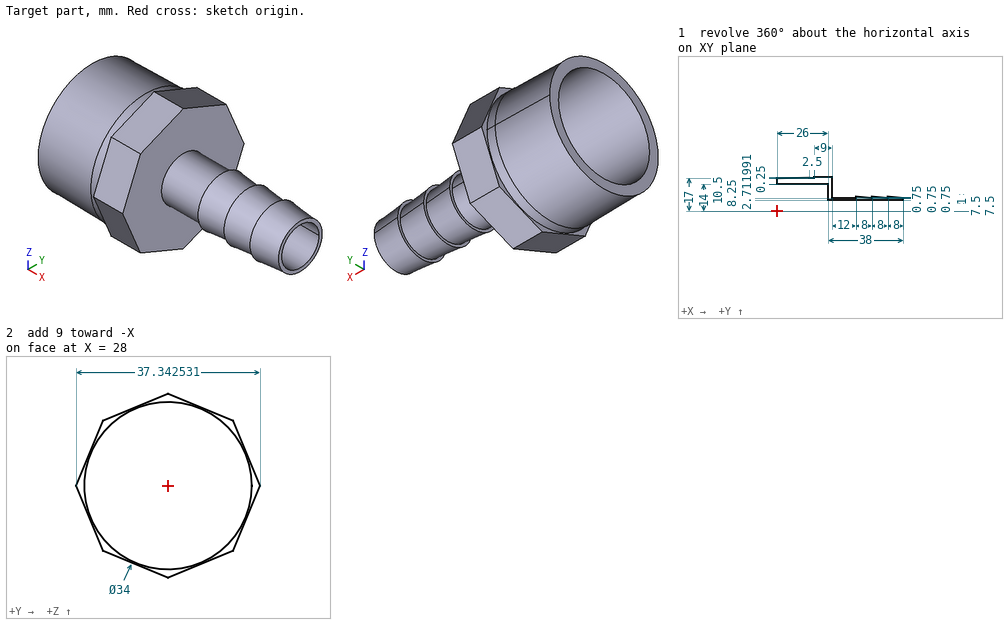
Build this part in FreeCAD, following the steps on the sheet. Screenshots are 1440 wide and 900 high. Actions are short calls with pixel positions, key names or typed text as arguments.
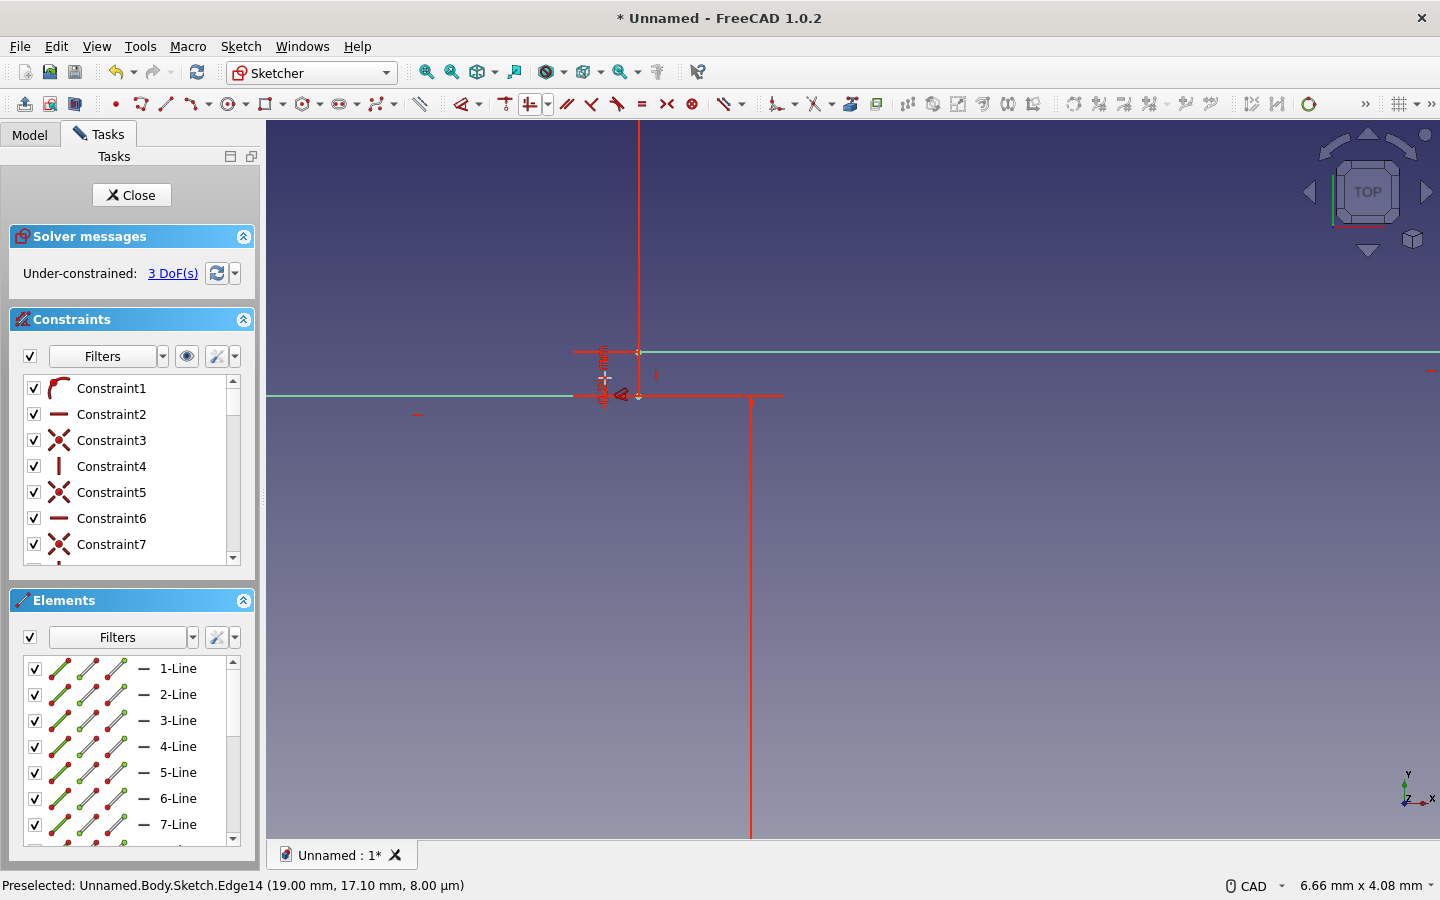
scroll(645, 389, down, 14)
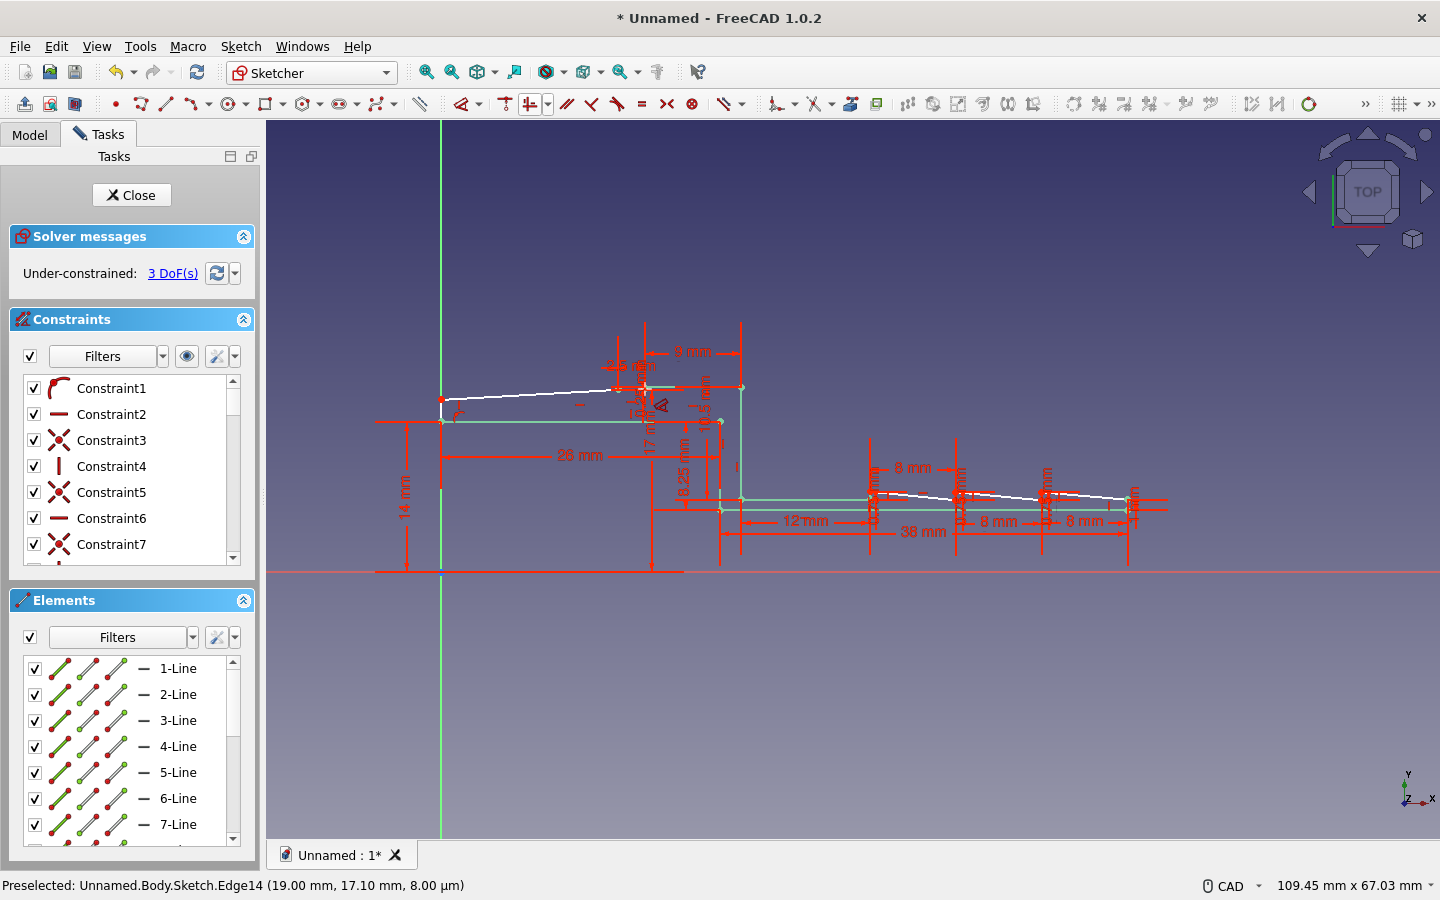
scroll(1042, 492, up, 3)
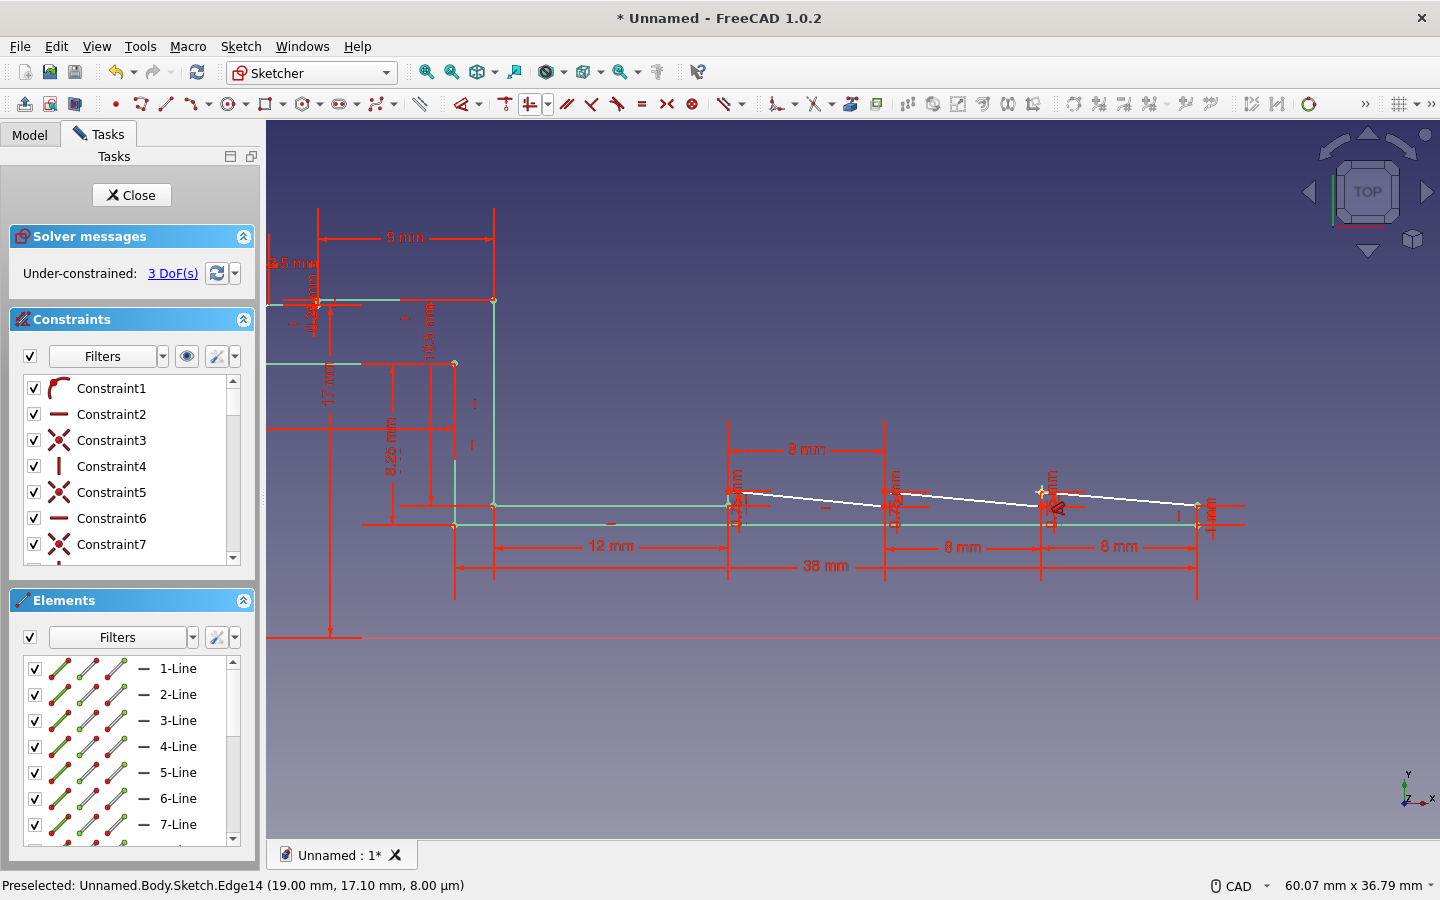
click(1041, 492)
click(1075, 598)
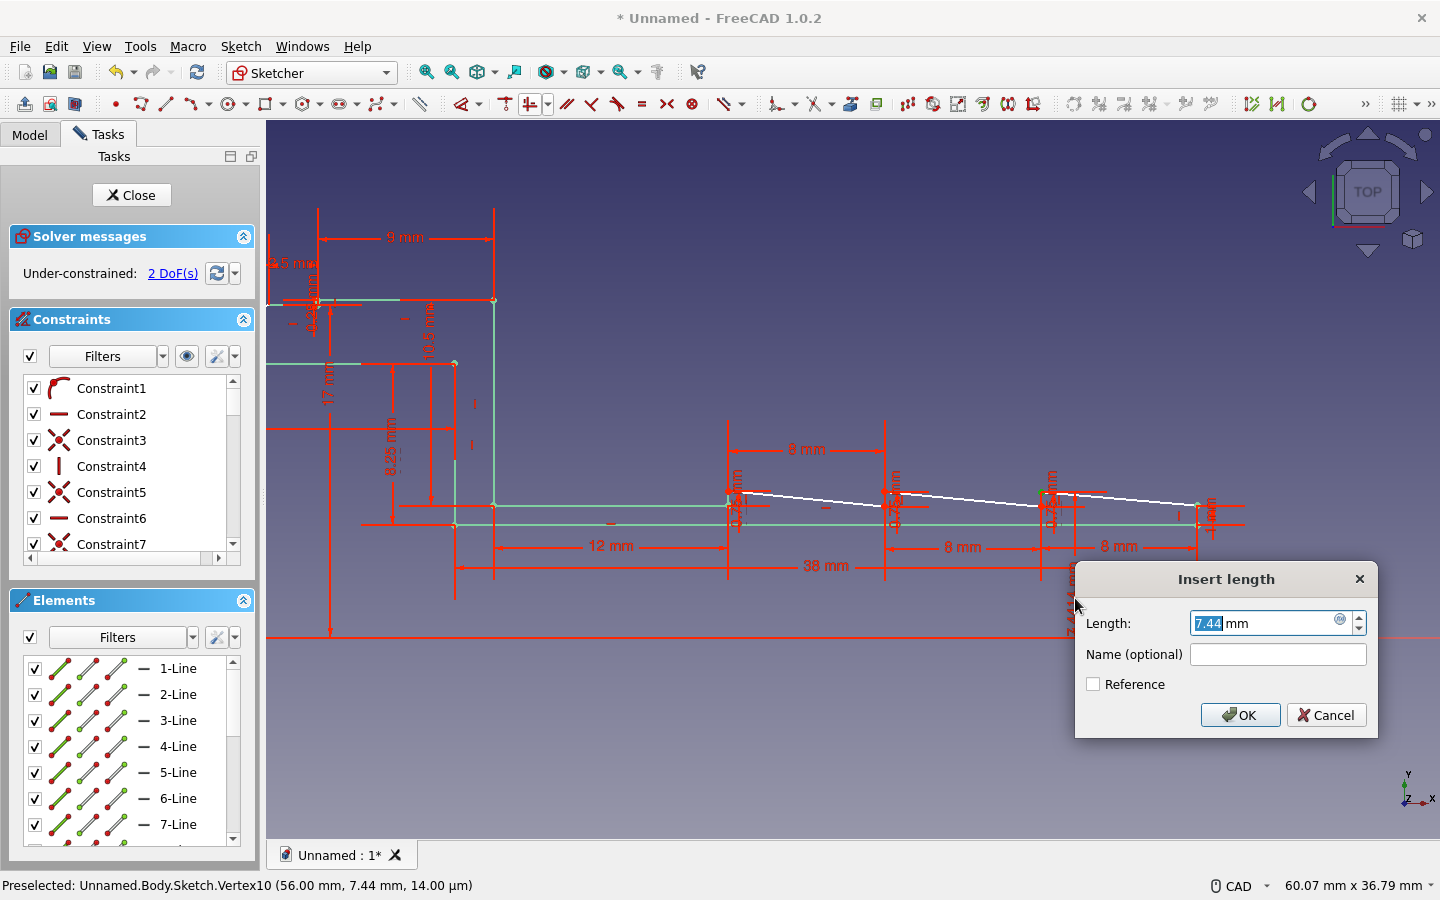
text(7.5)
key(Return)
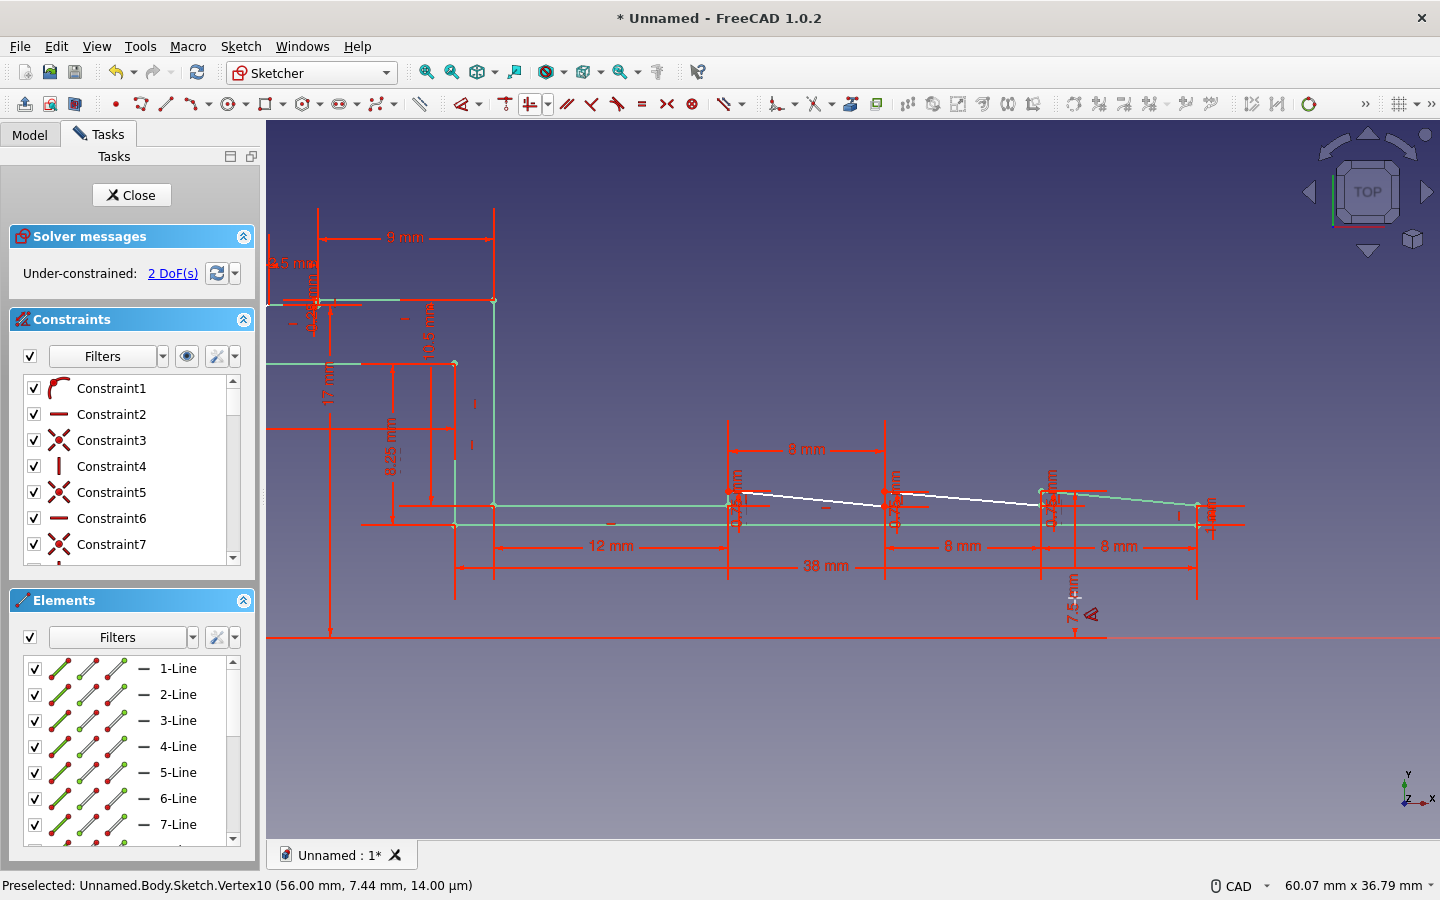
click(885, 492)
click(919, 598)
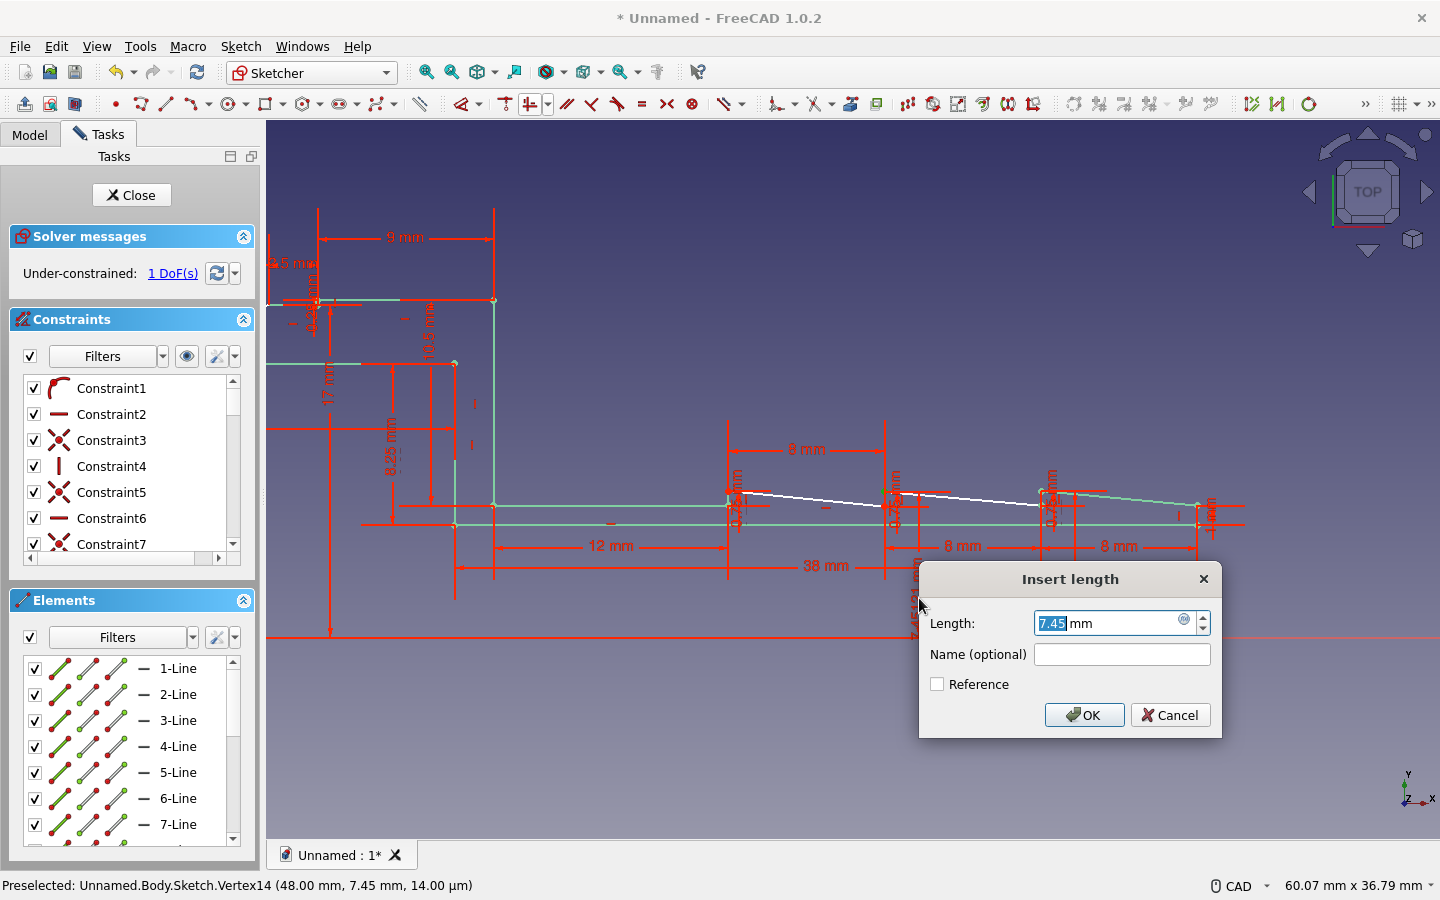
text(7.5)
key(Return)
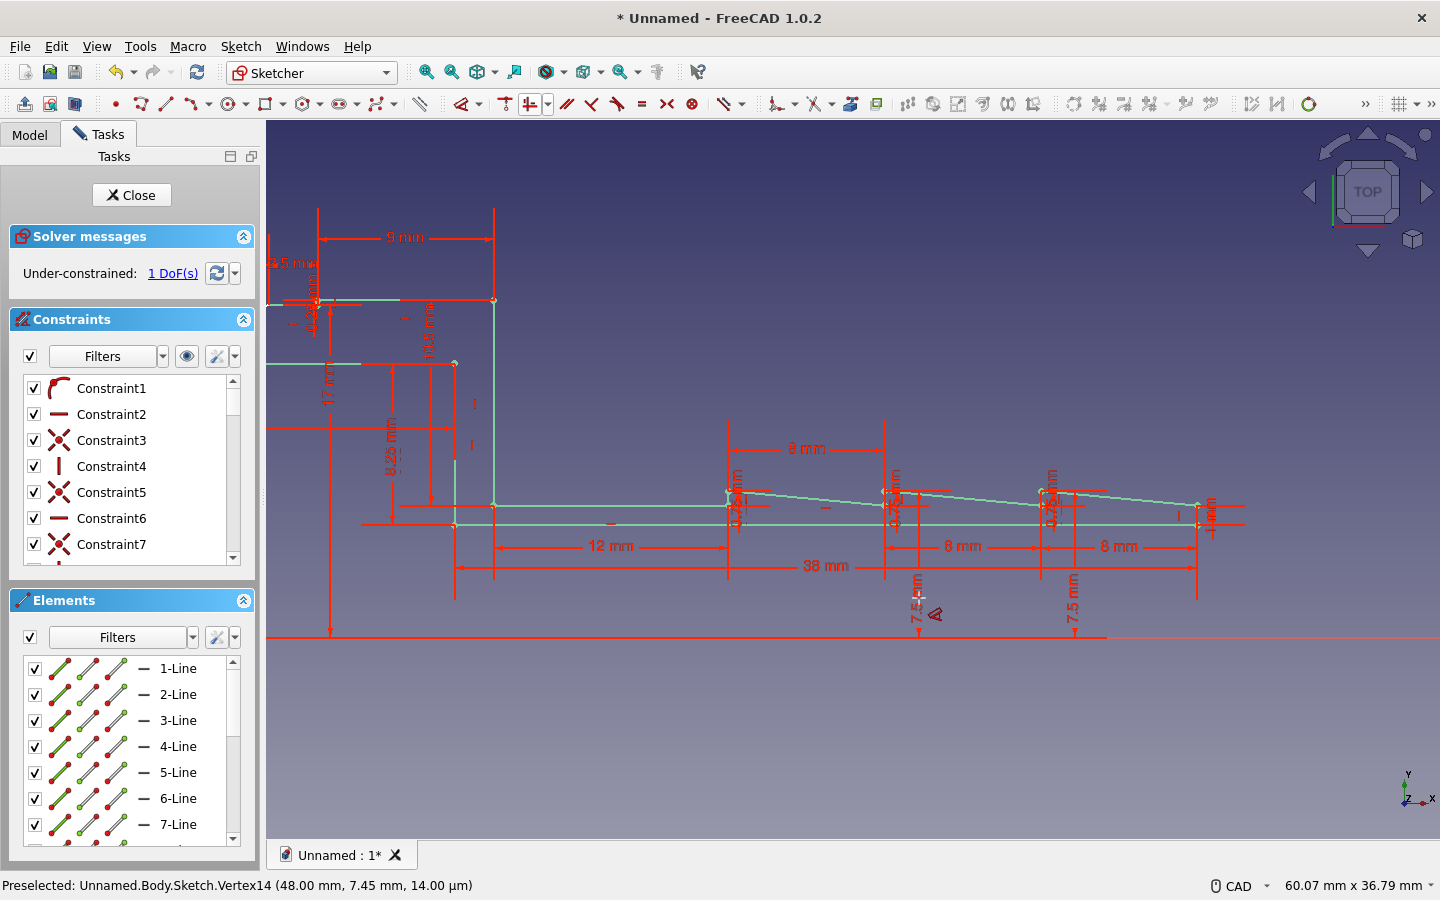
scroll(1043, 492, down, 3)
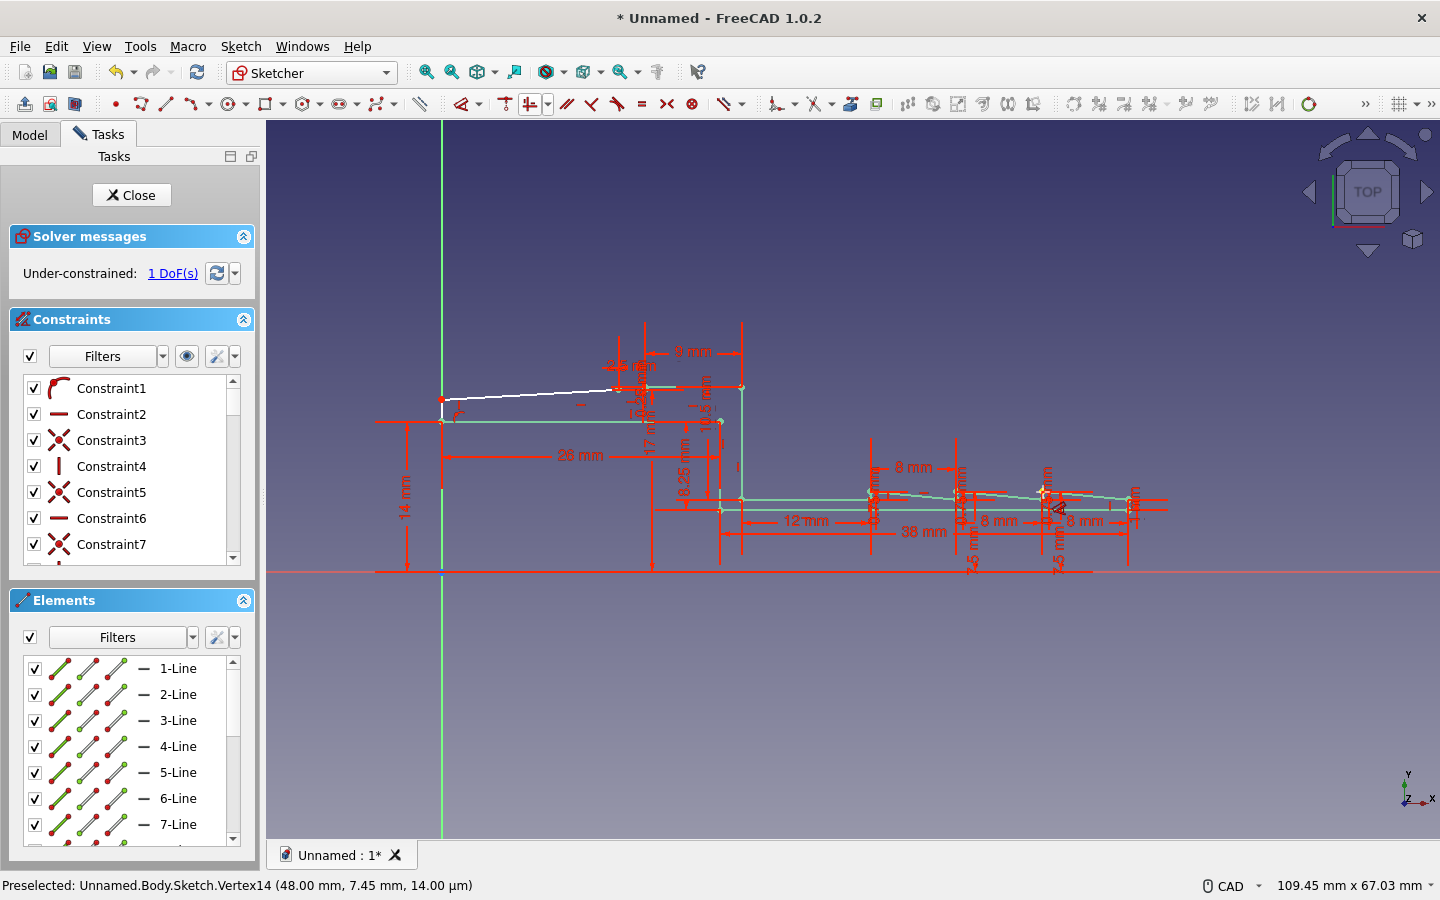
scroll(442, 407, up, 4)